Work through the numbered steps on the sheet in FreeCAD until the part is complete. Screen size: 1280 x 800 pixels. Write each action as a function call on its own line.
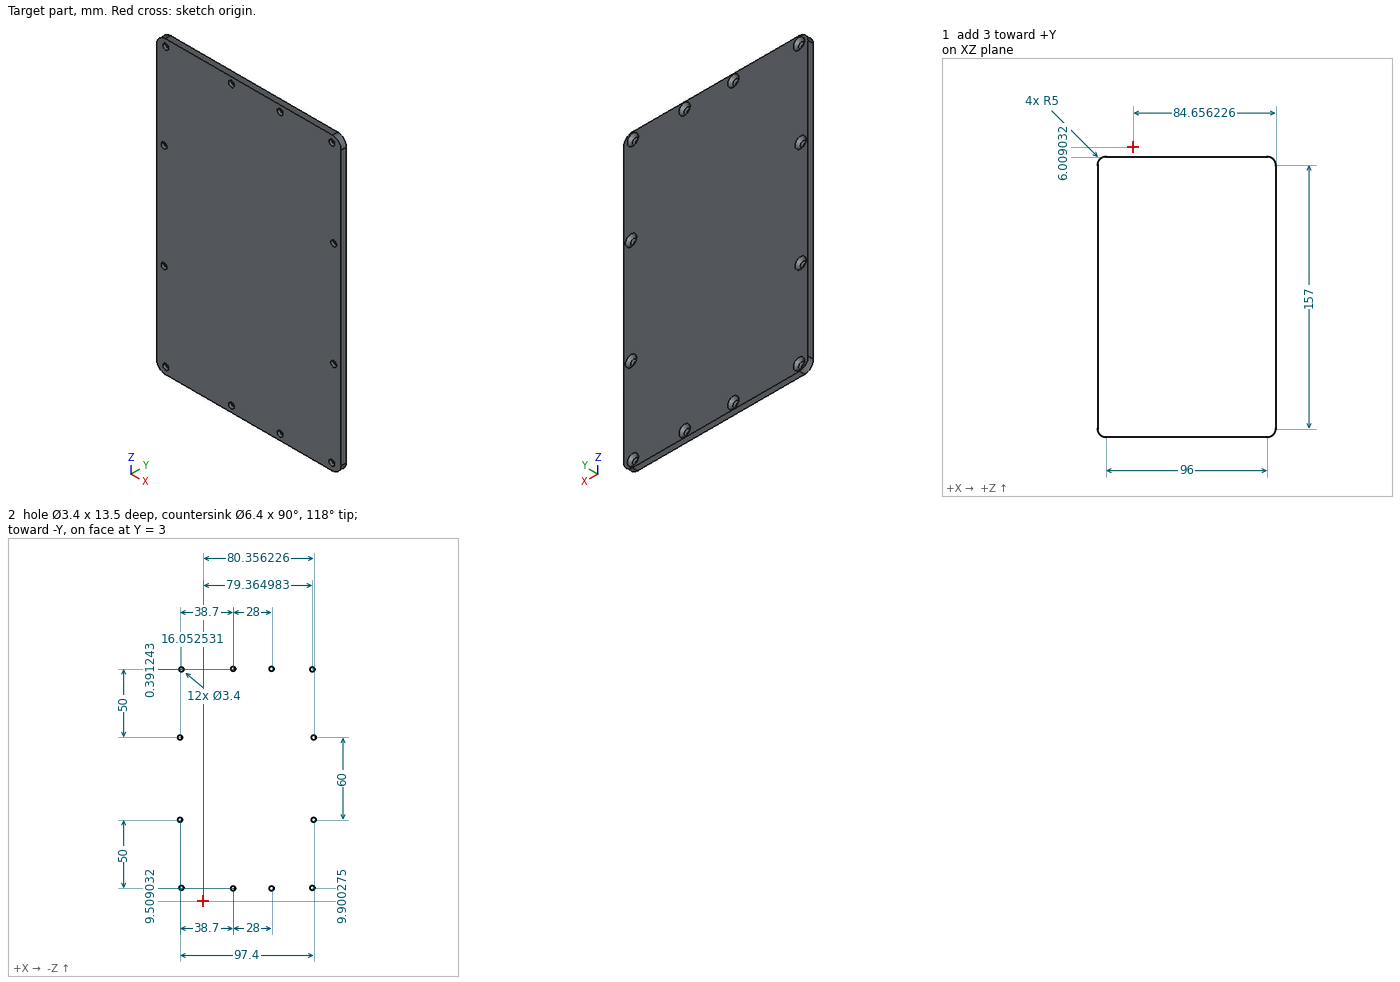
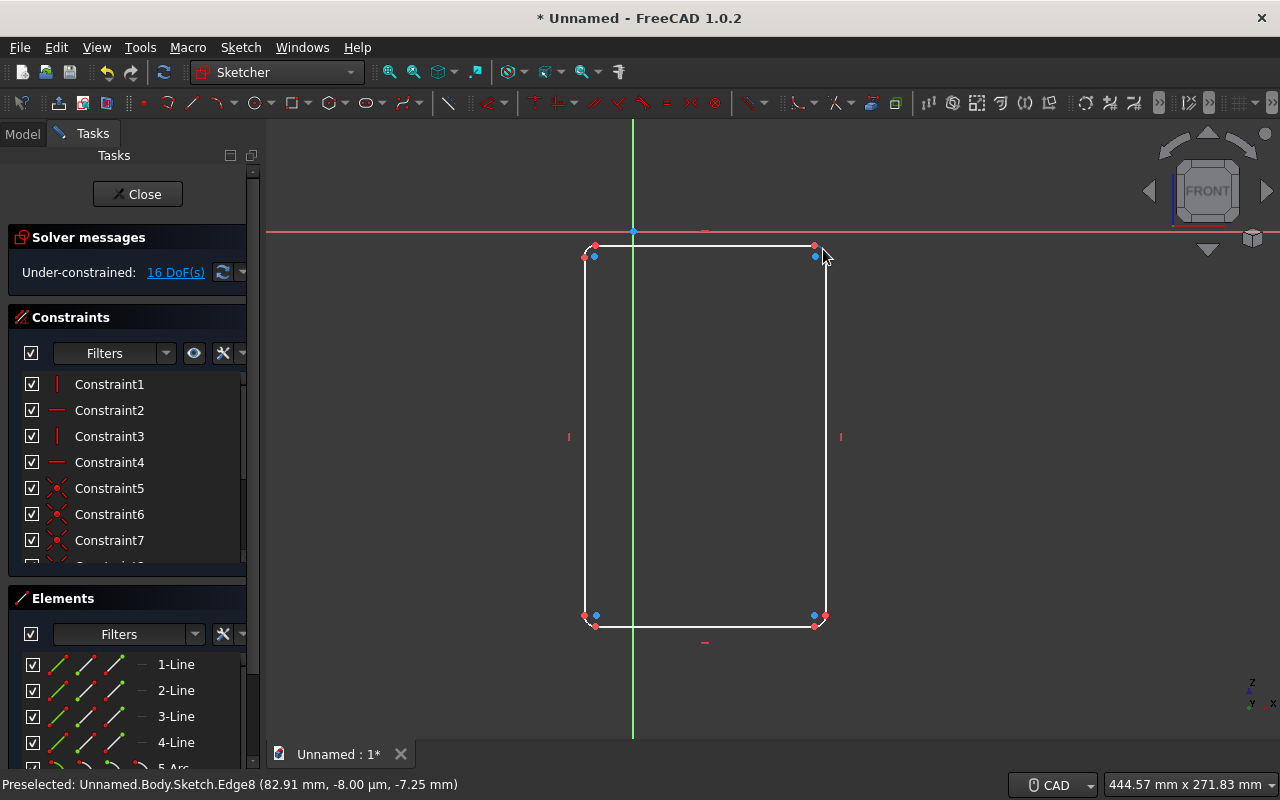
click(826, 329)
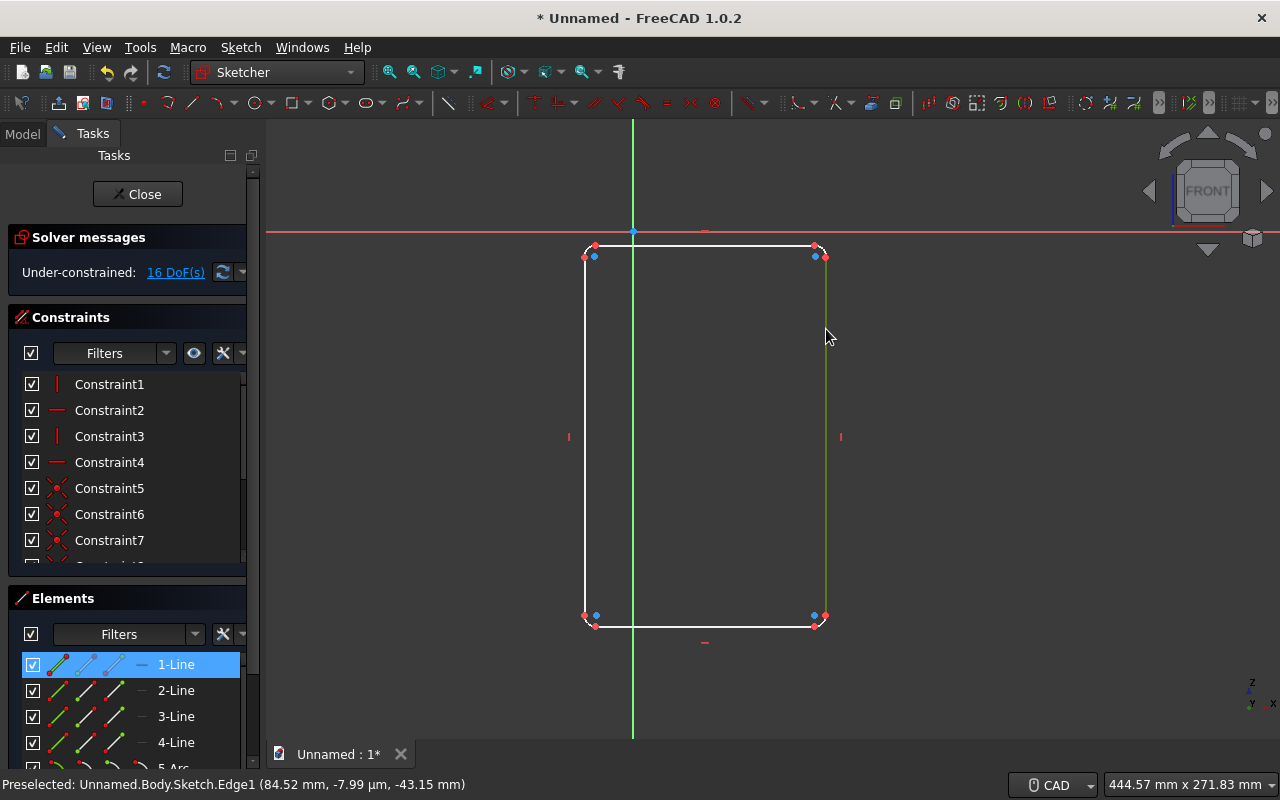
scroll(822, 623, up, 3)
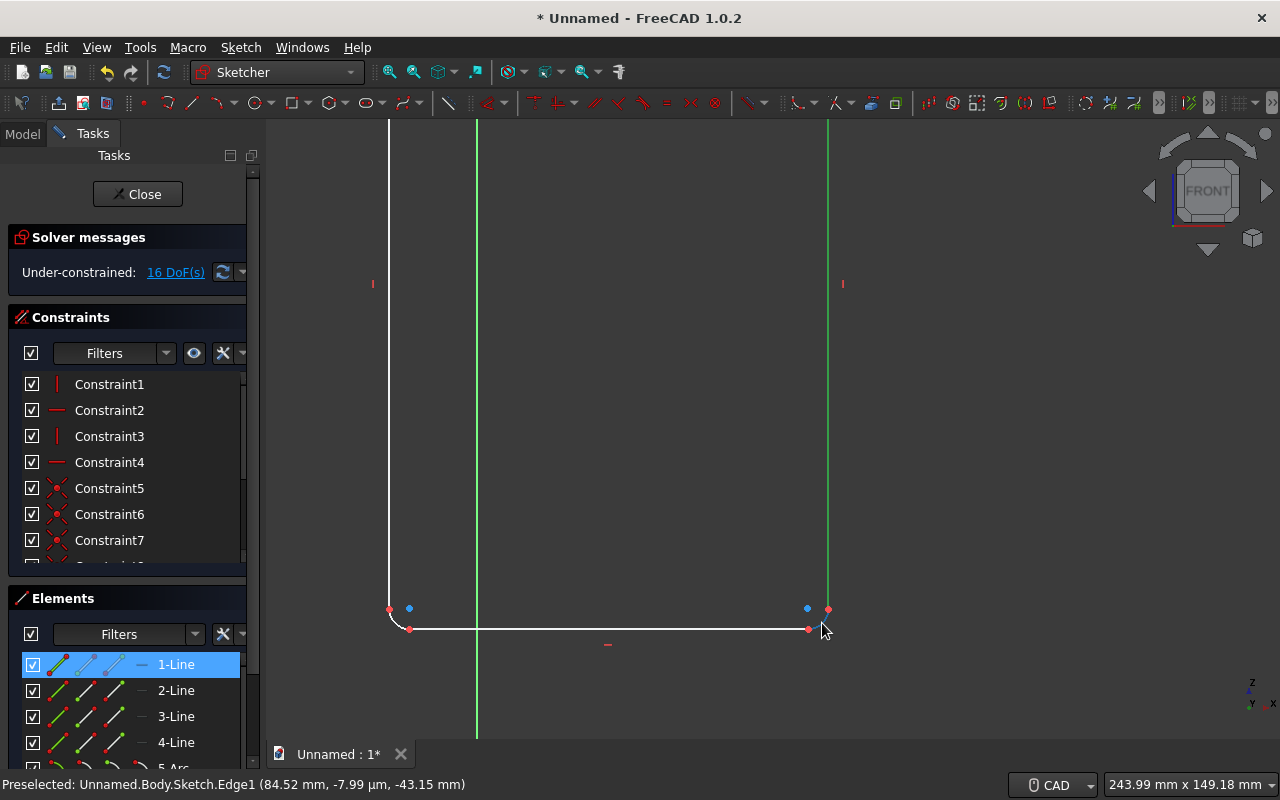
click(822, 623)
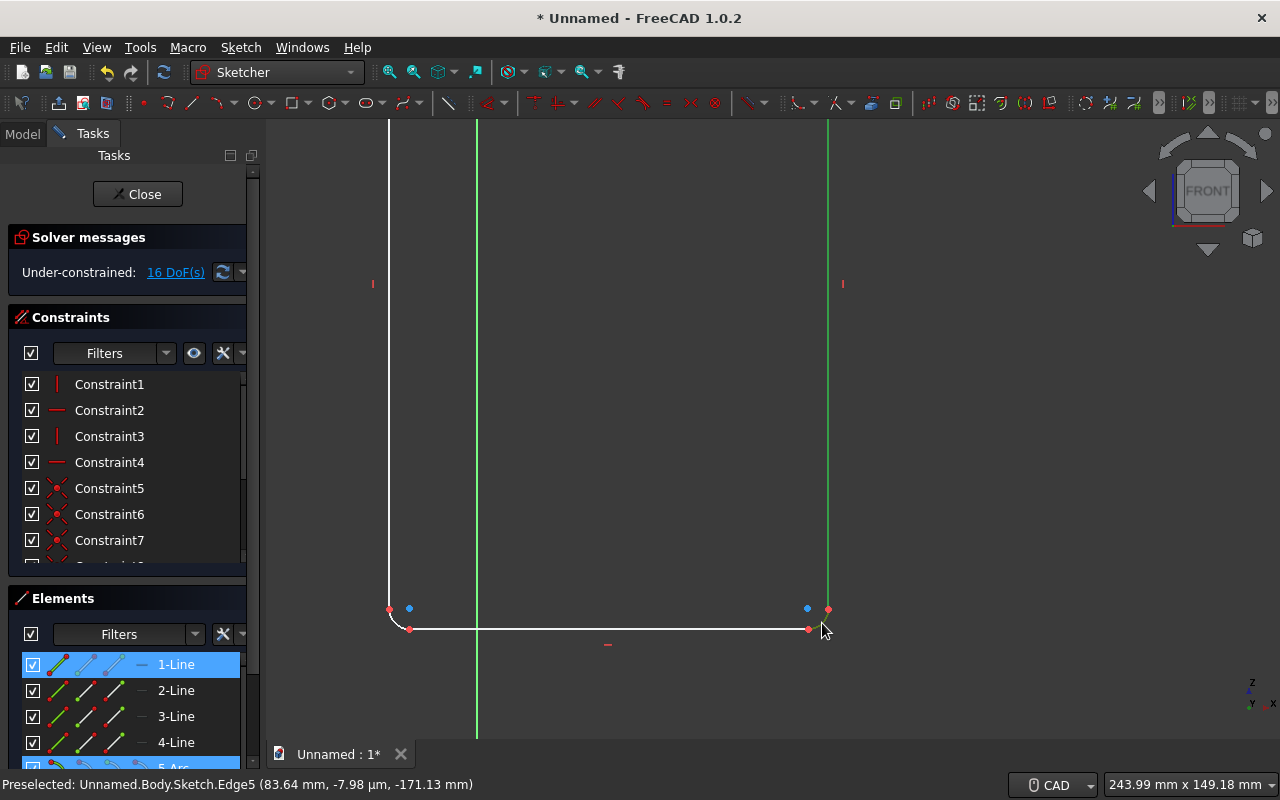
click(644, 104)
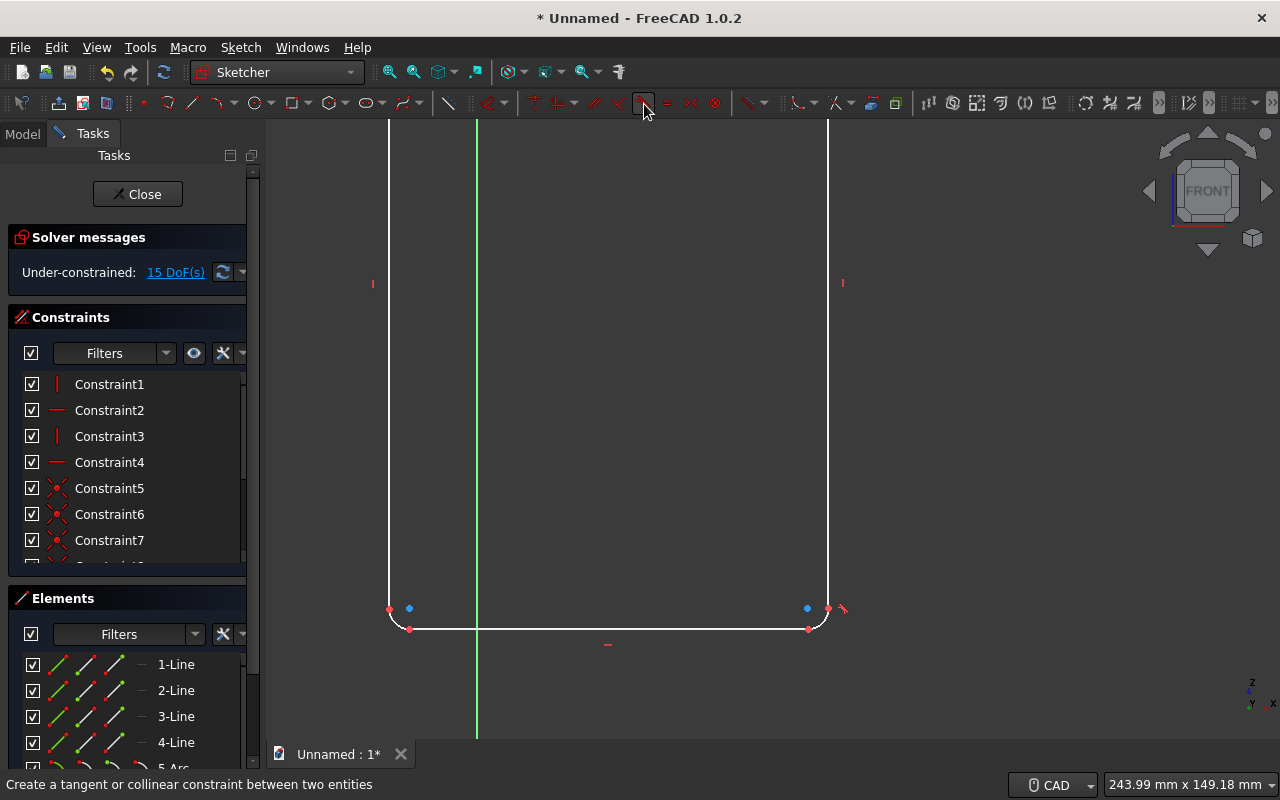
click(828, 152)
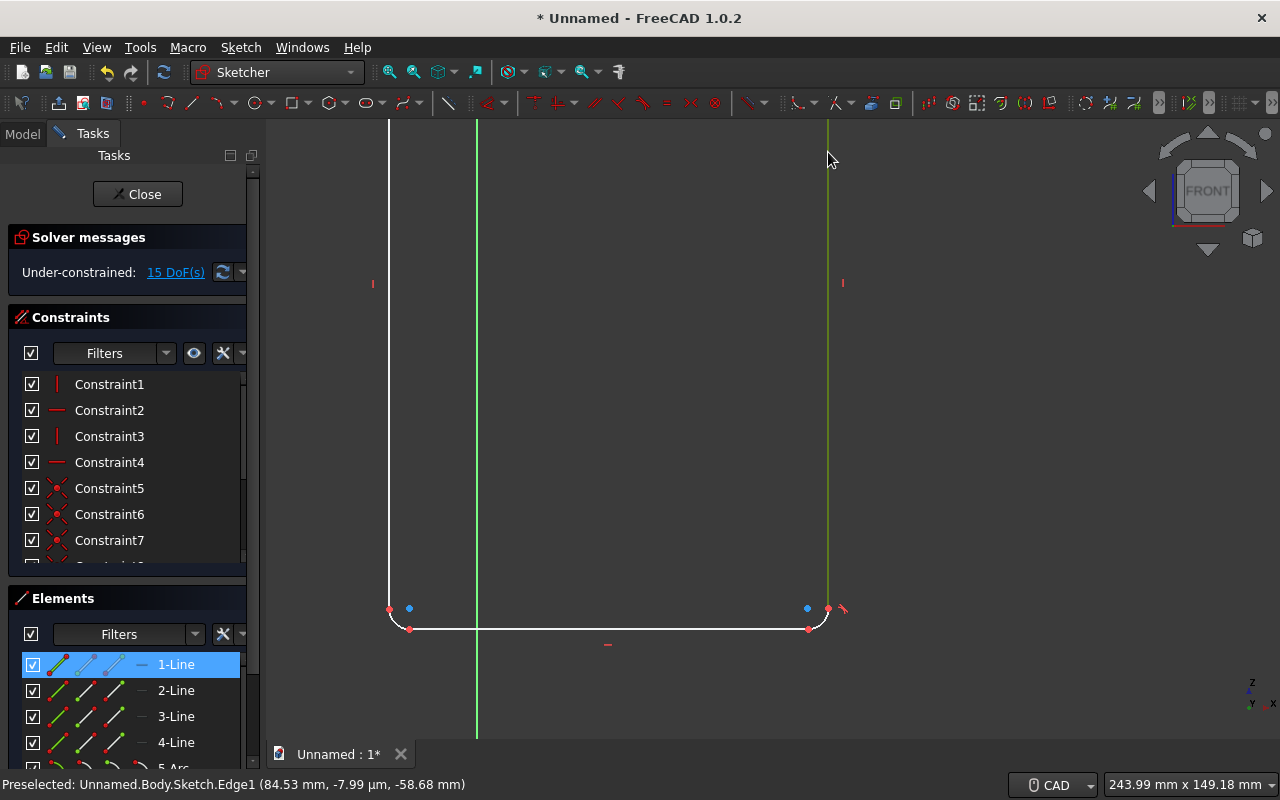
scroll(821, 624, down, 3)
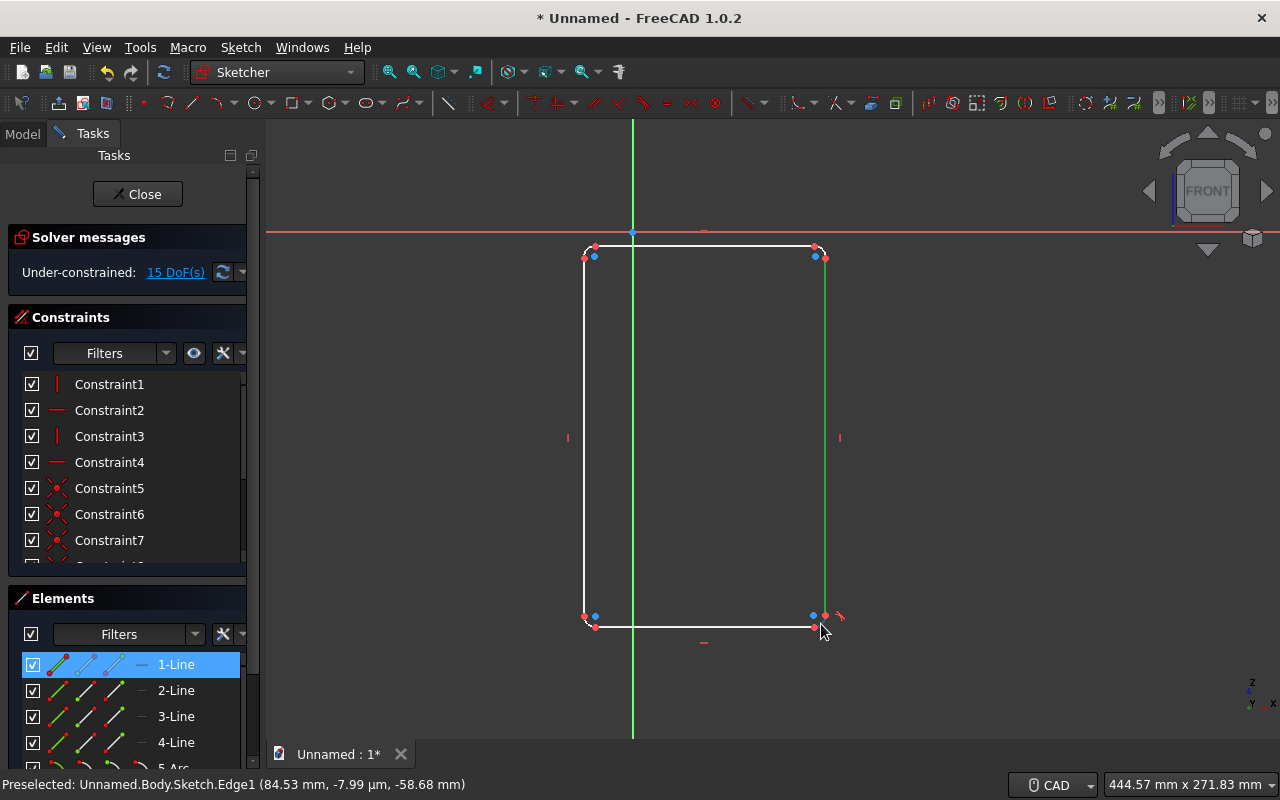
scroll(825, 253, up, 5)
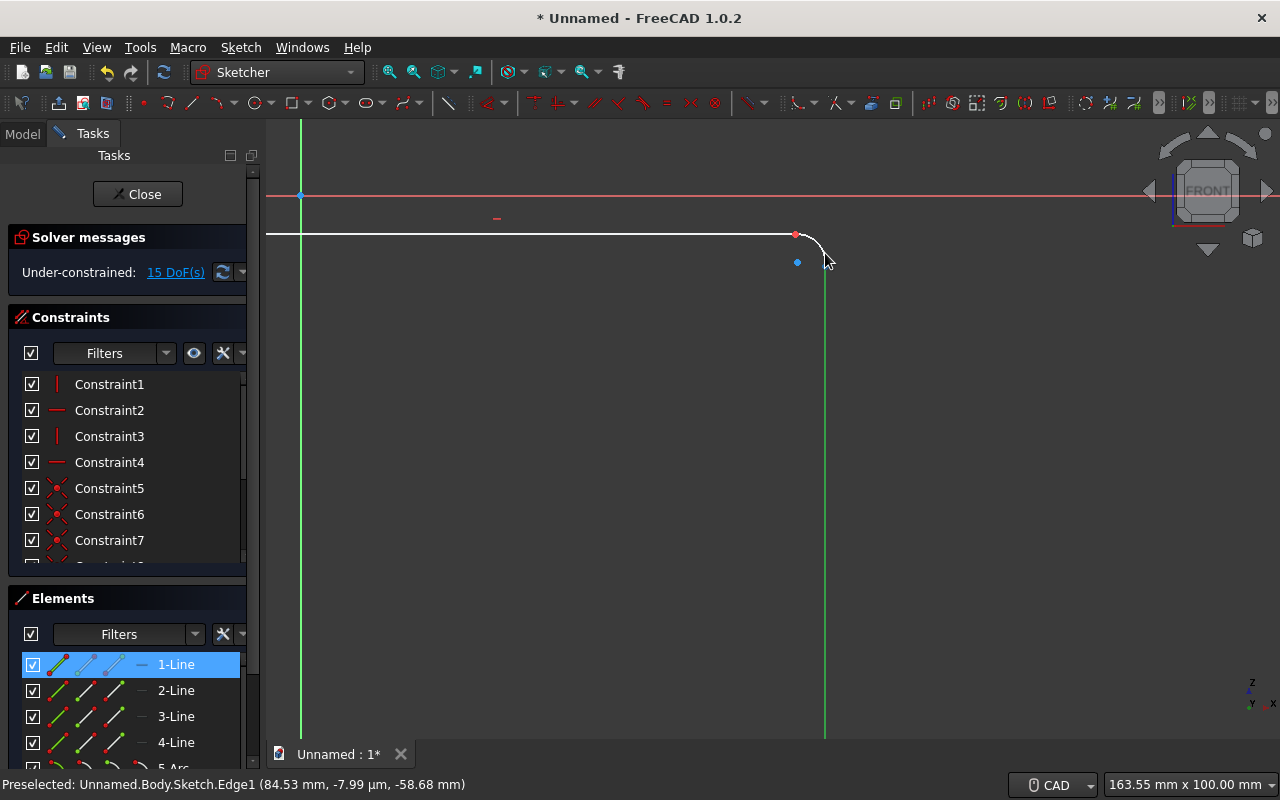
click(823, 252)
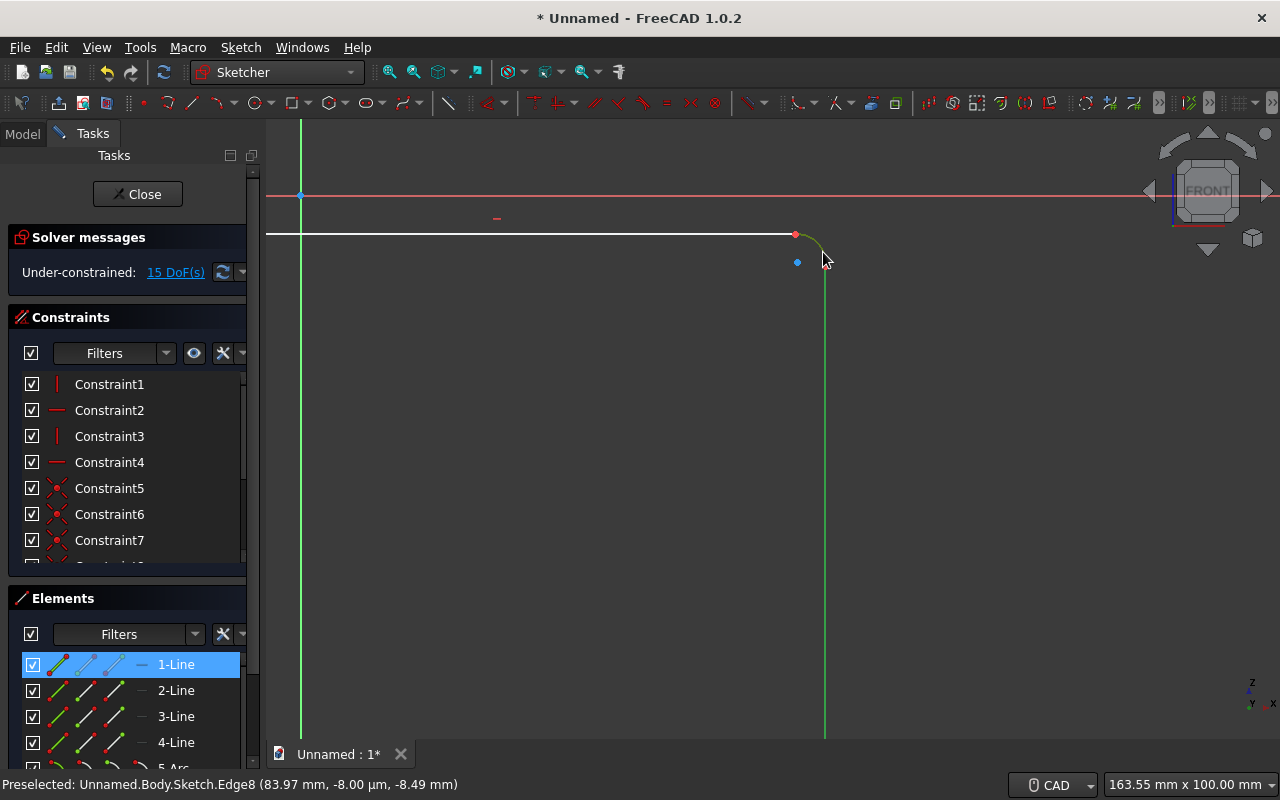
click(644, 104)